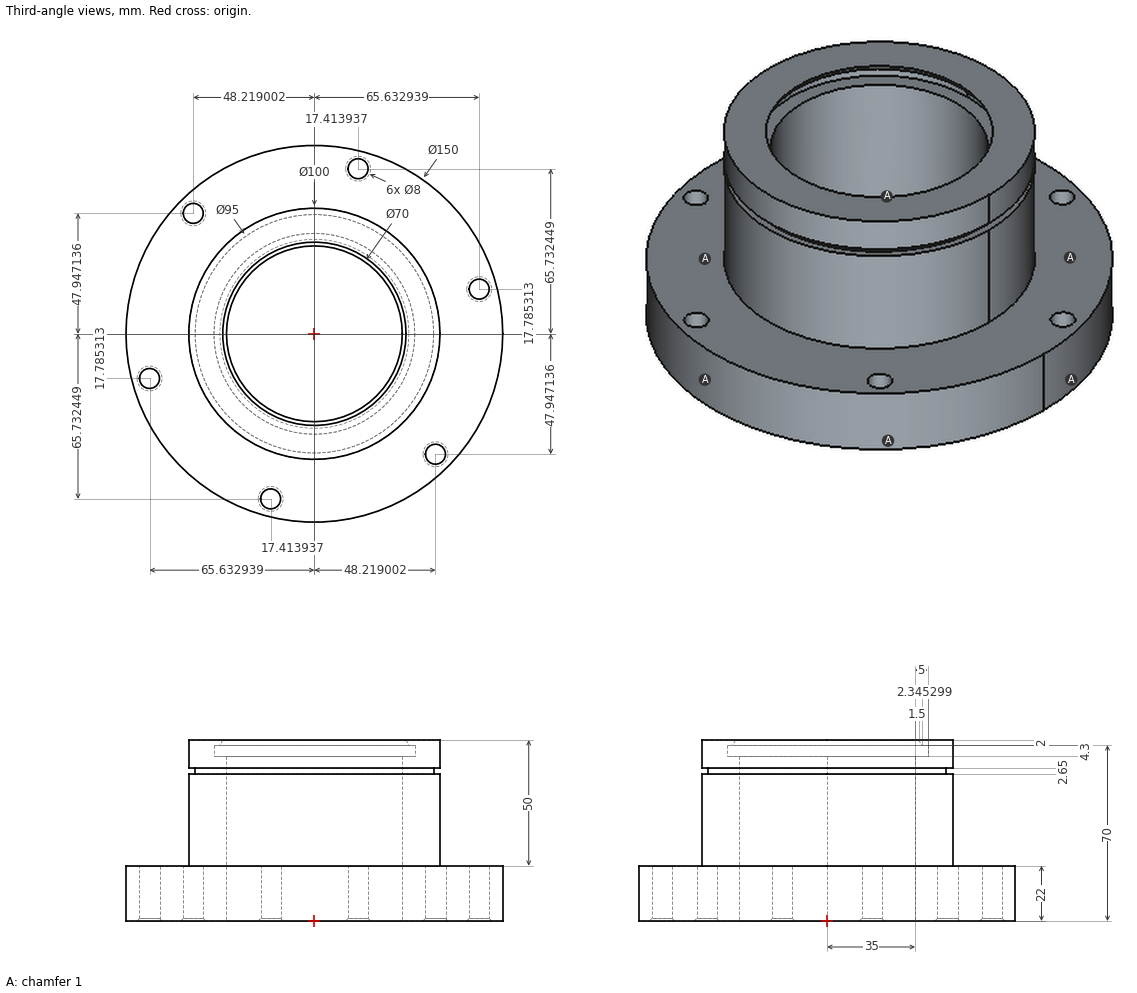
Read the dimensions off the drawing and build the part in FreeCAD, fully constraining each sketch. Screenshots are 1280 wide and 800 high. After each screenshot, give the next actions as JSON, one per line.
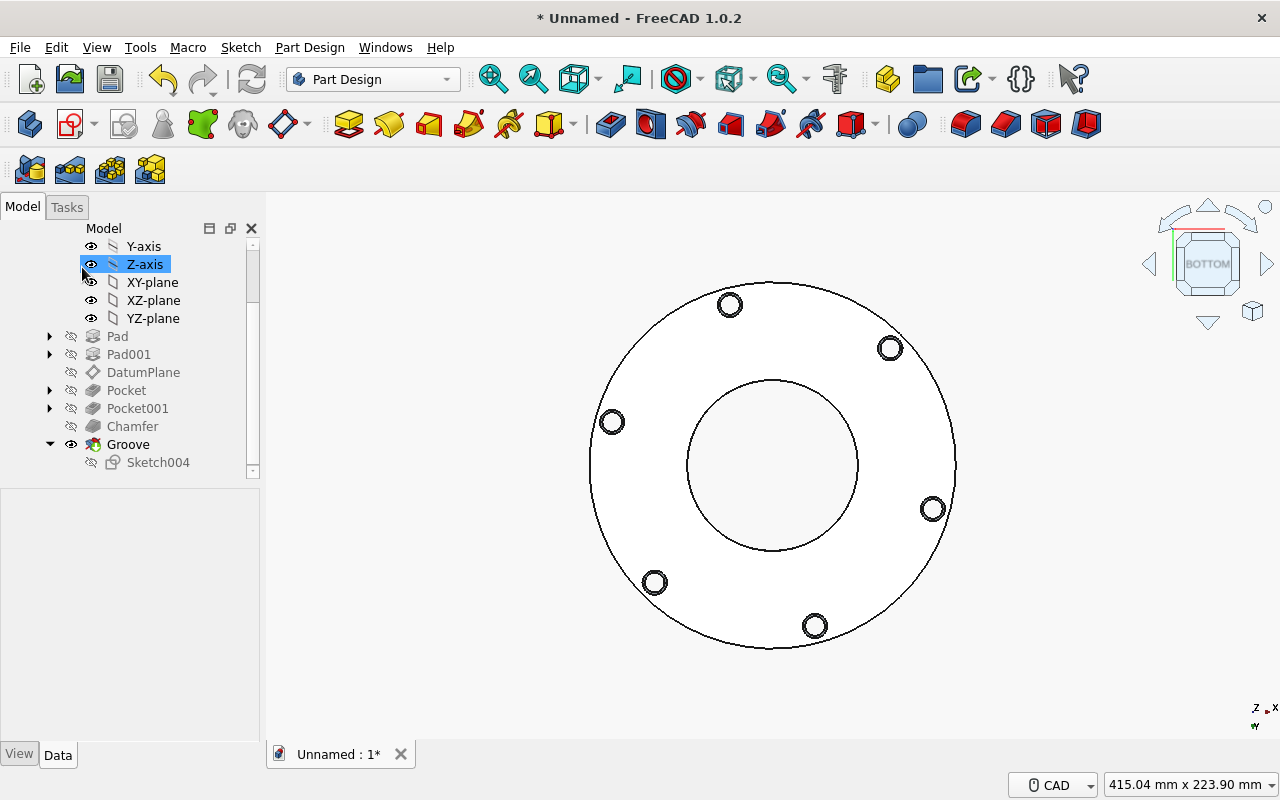
{"action": "key", "text": "0"}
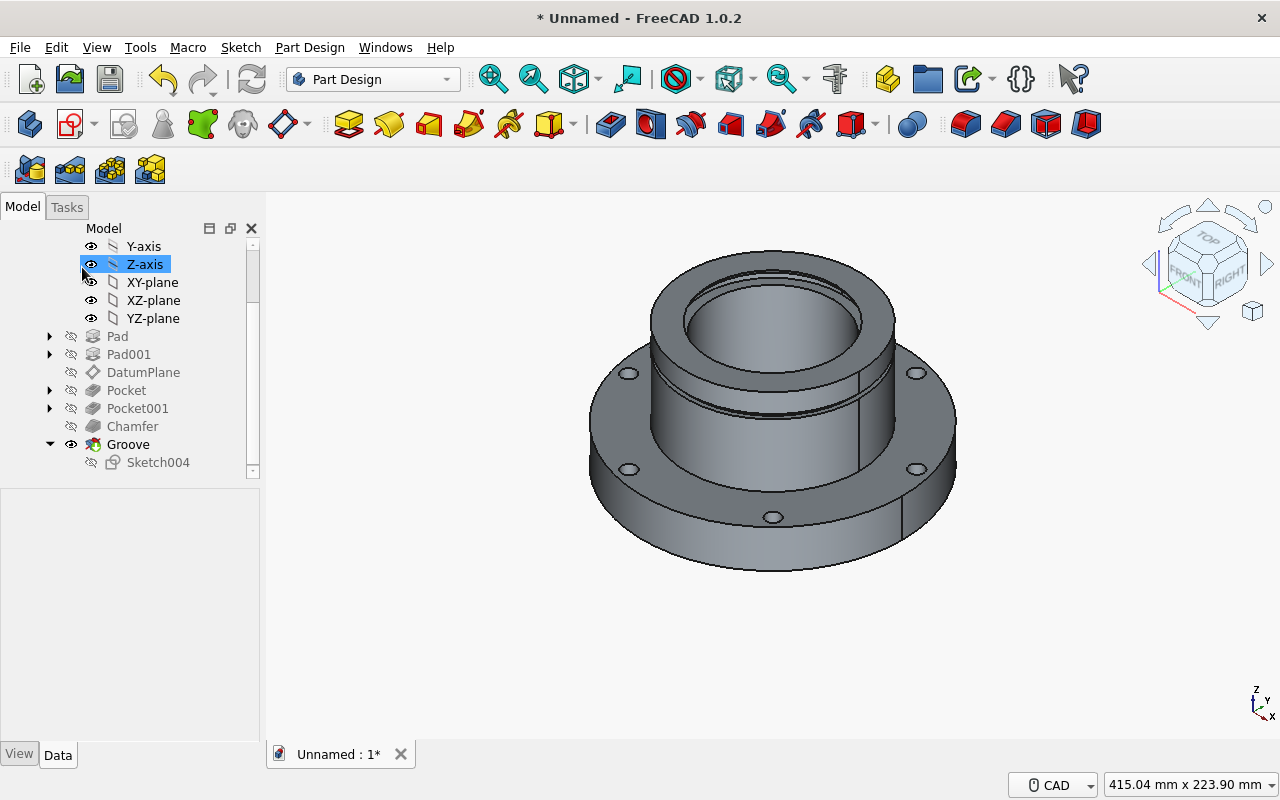
{"action": "left_click", "coordinate": [494, 80]}